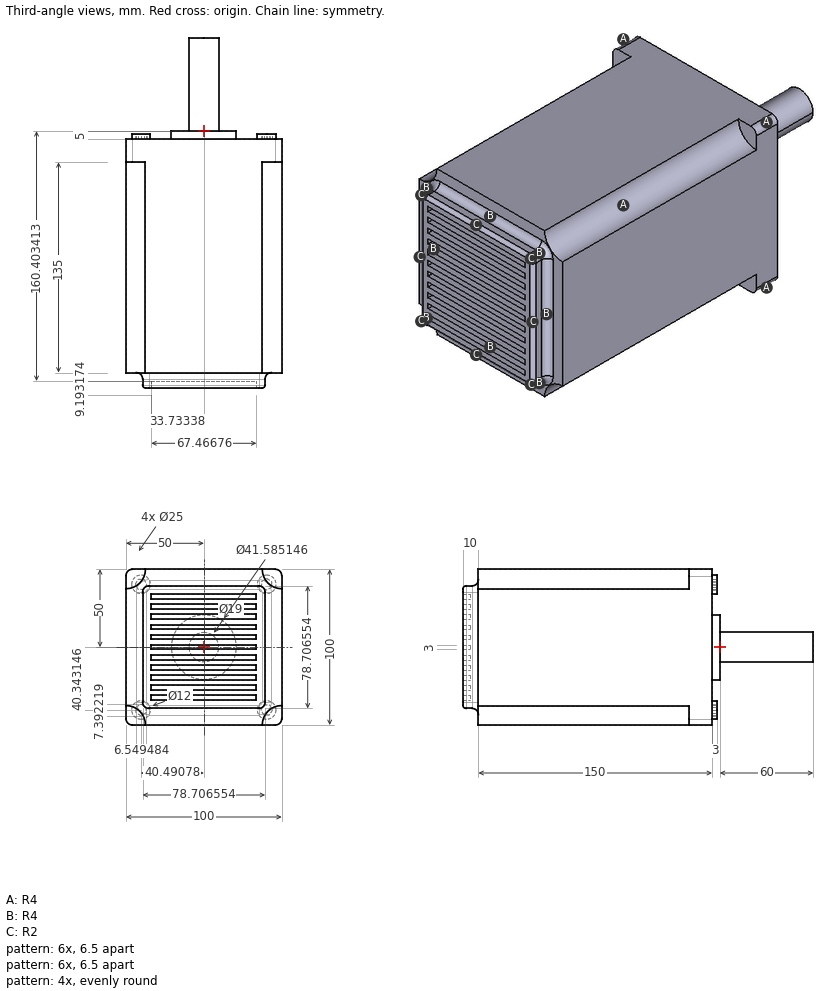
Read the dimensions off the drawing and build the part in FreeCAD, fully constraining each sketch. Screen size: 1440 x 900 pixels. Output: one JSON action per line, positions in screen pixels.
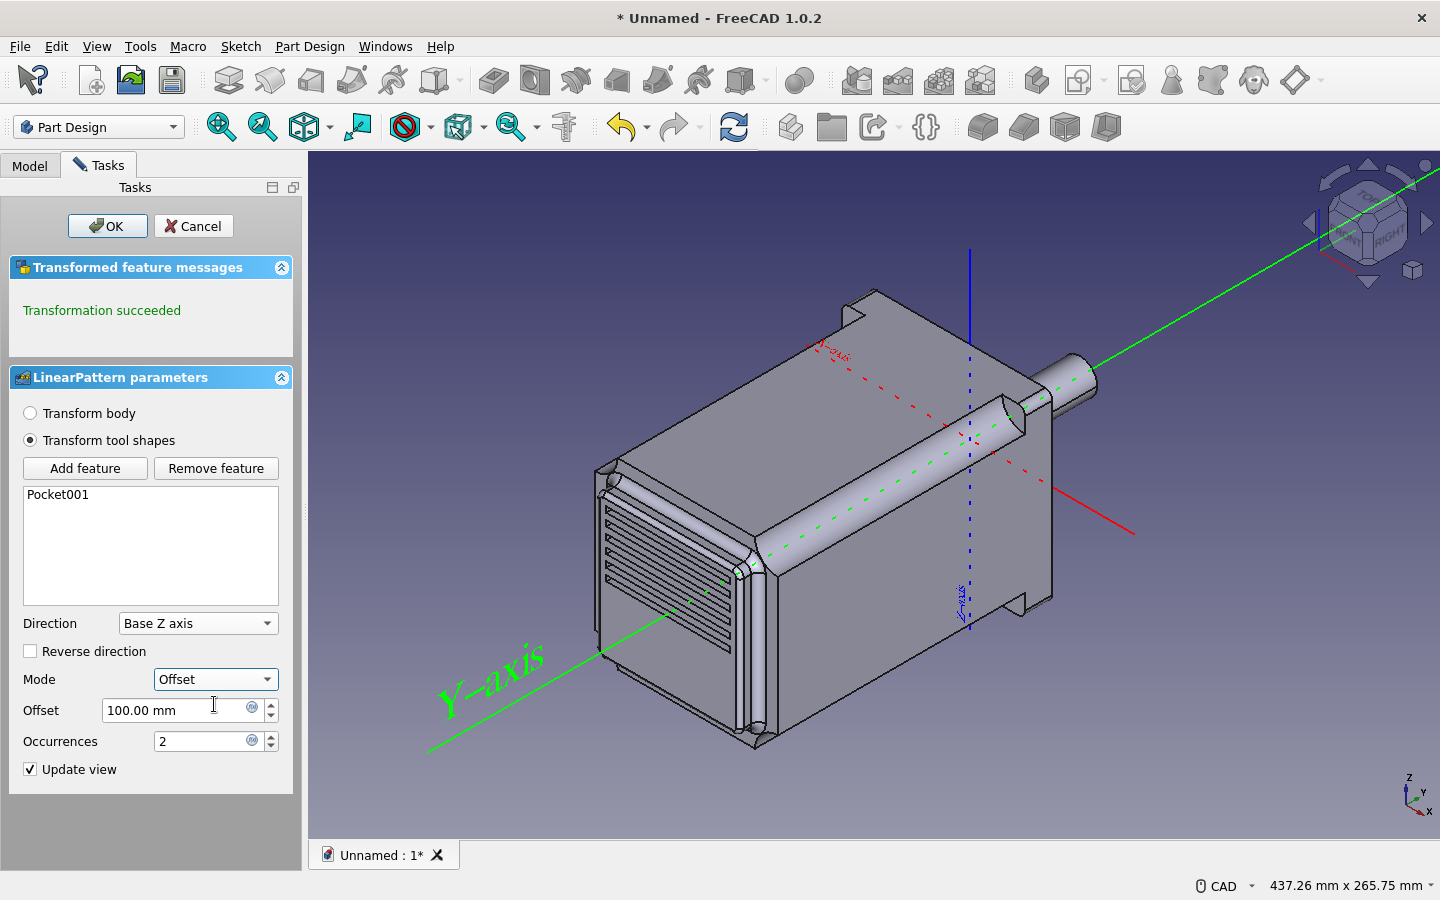
{"action": "triple_click", "coordinate": [184, 710]}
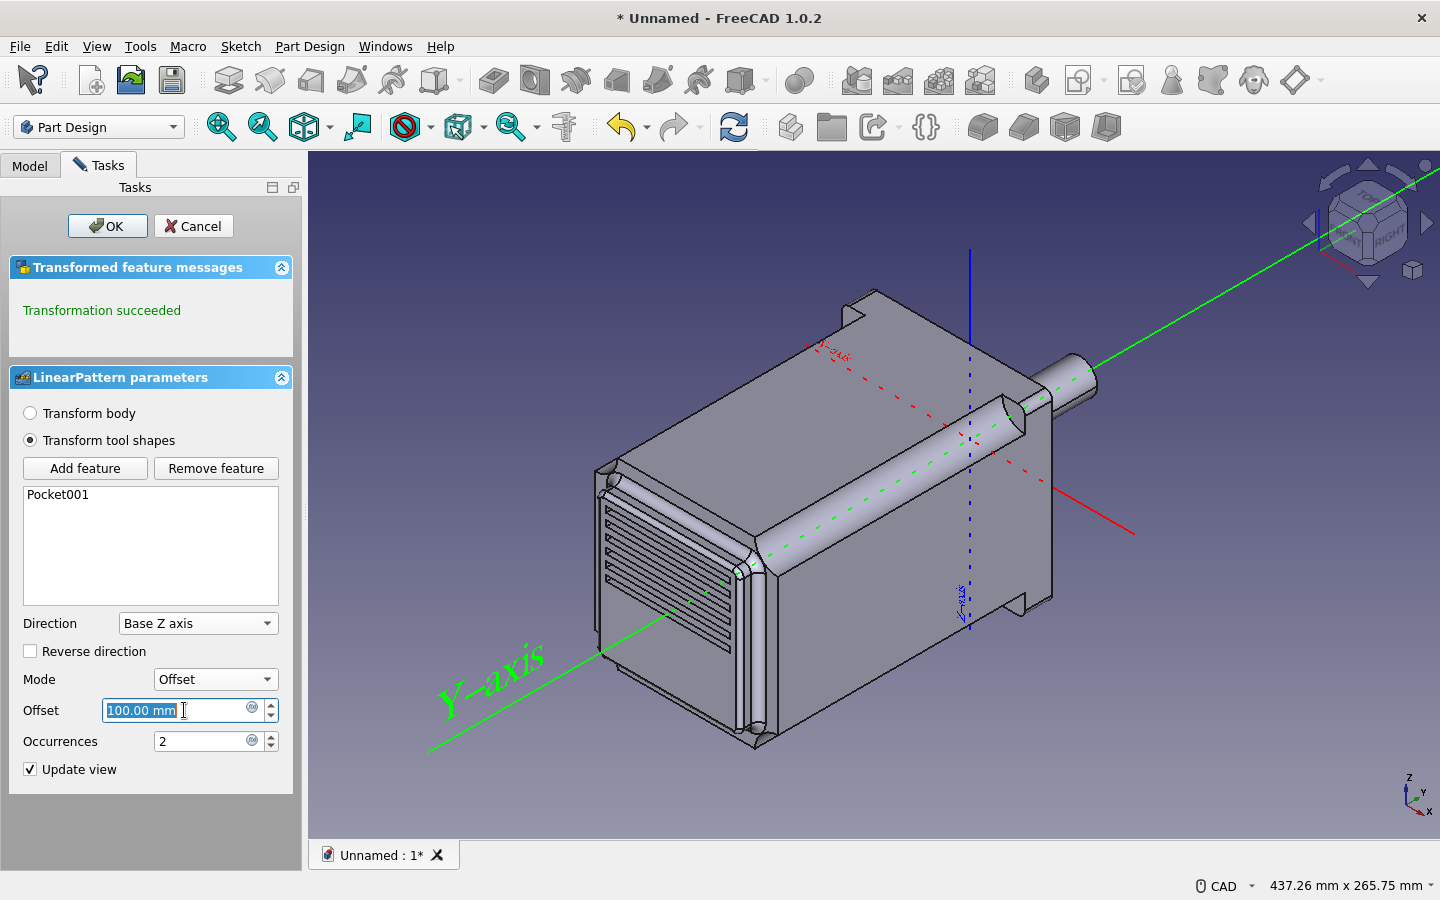
{"action": "type", "text": "6.5"}
{"action": "key", "text": "Tab"}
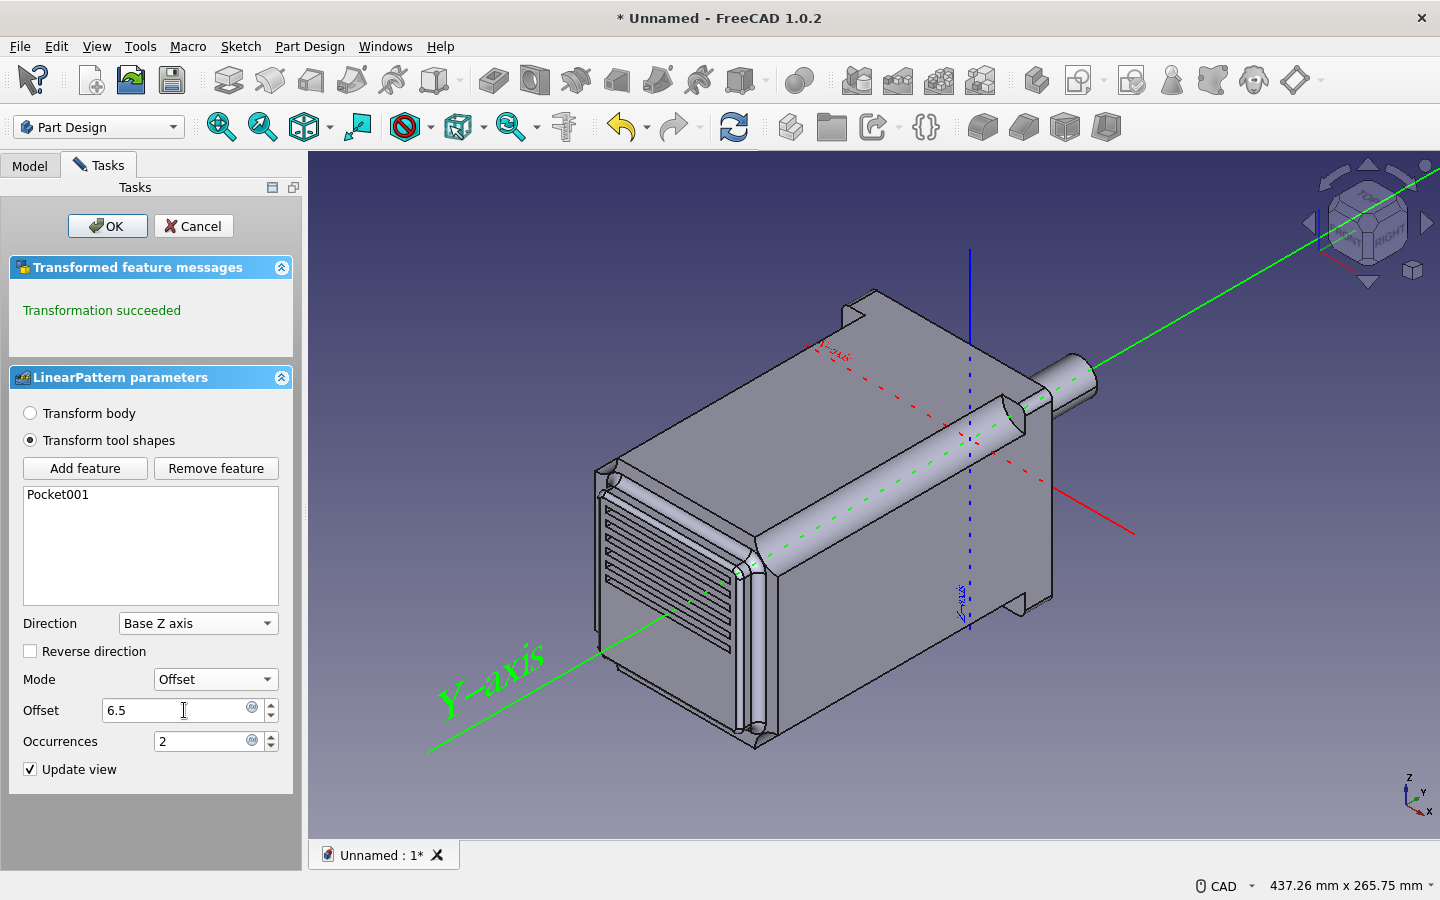
{"action": "triple_click", "coordinate": [210, 742]}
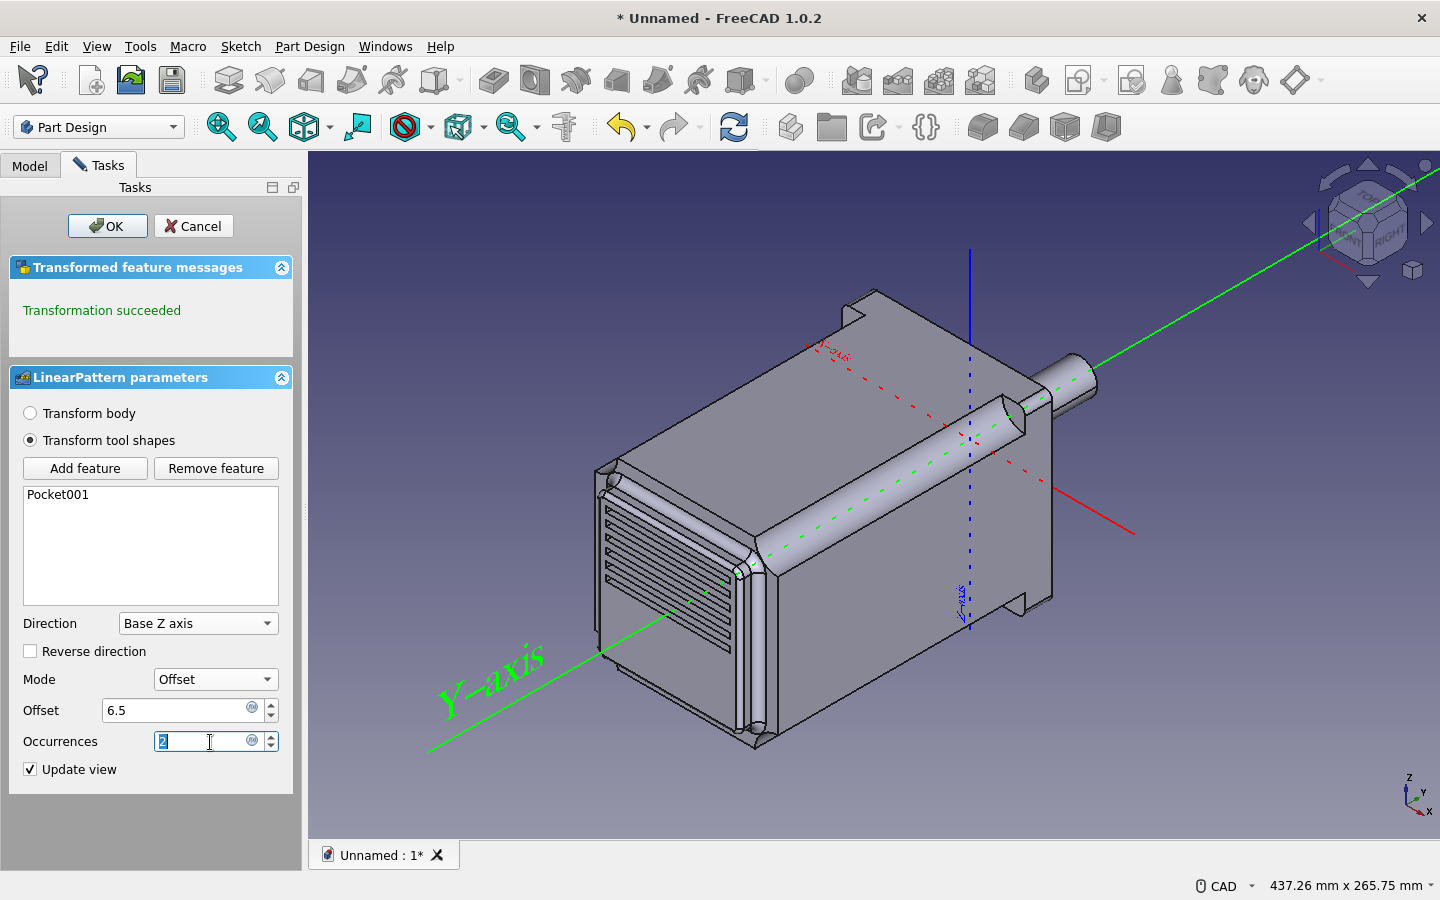
{"action": "type", "text": "6"}
{"action": "key", "text": "Tab"}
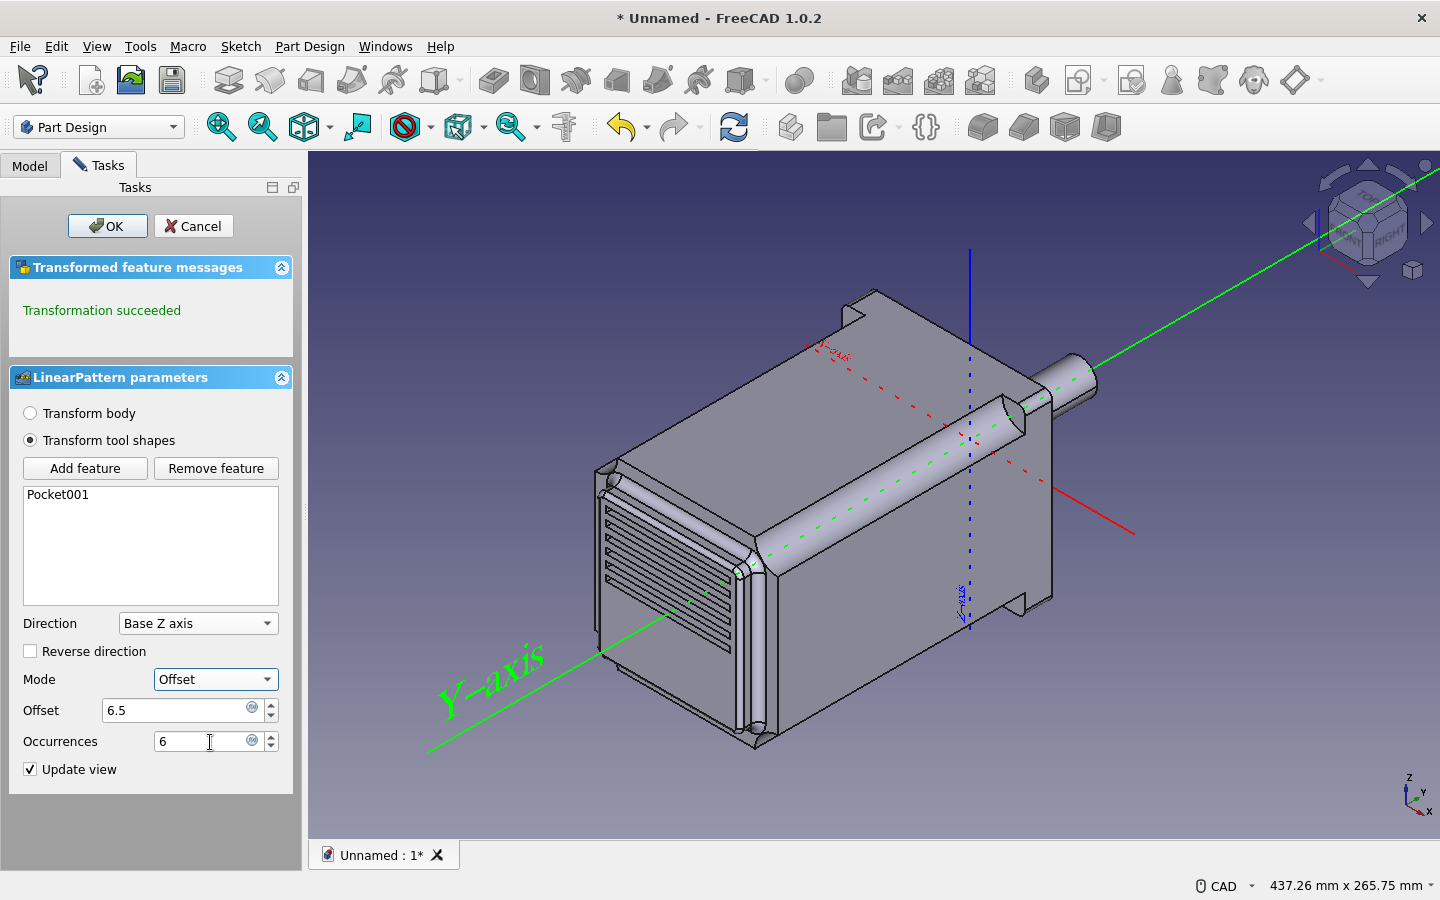
{"action": "left_click", "coordinate": [31, 651]}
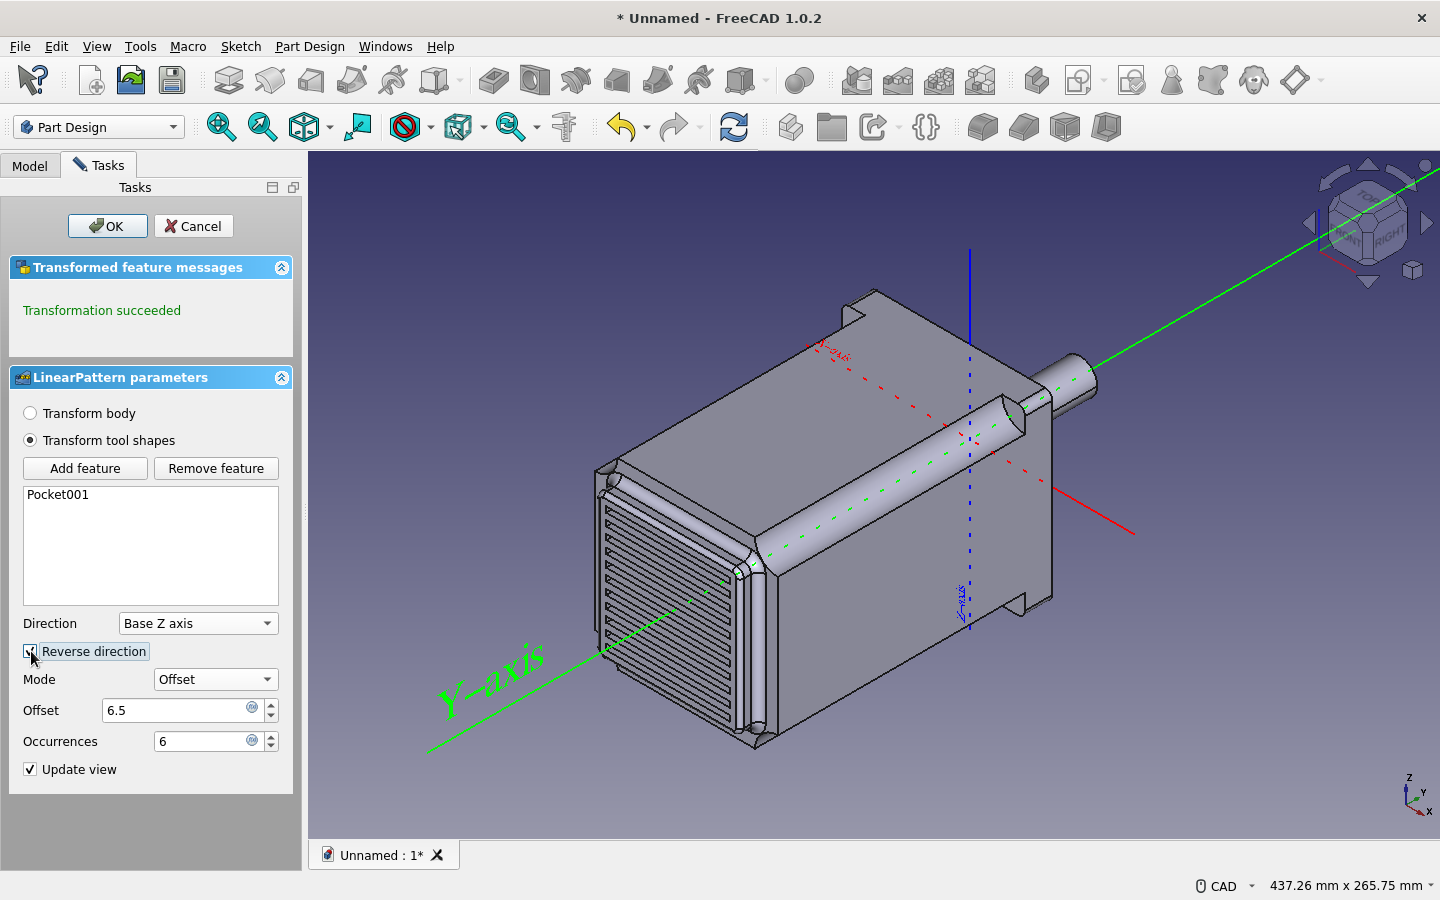
{"action": "left_click", "coordinate": [108, 226]}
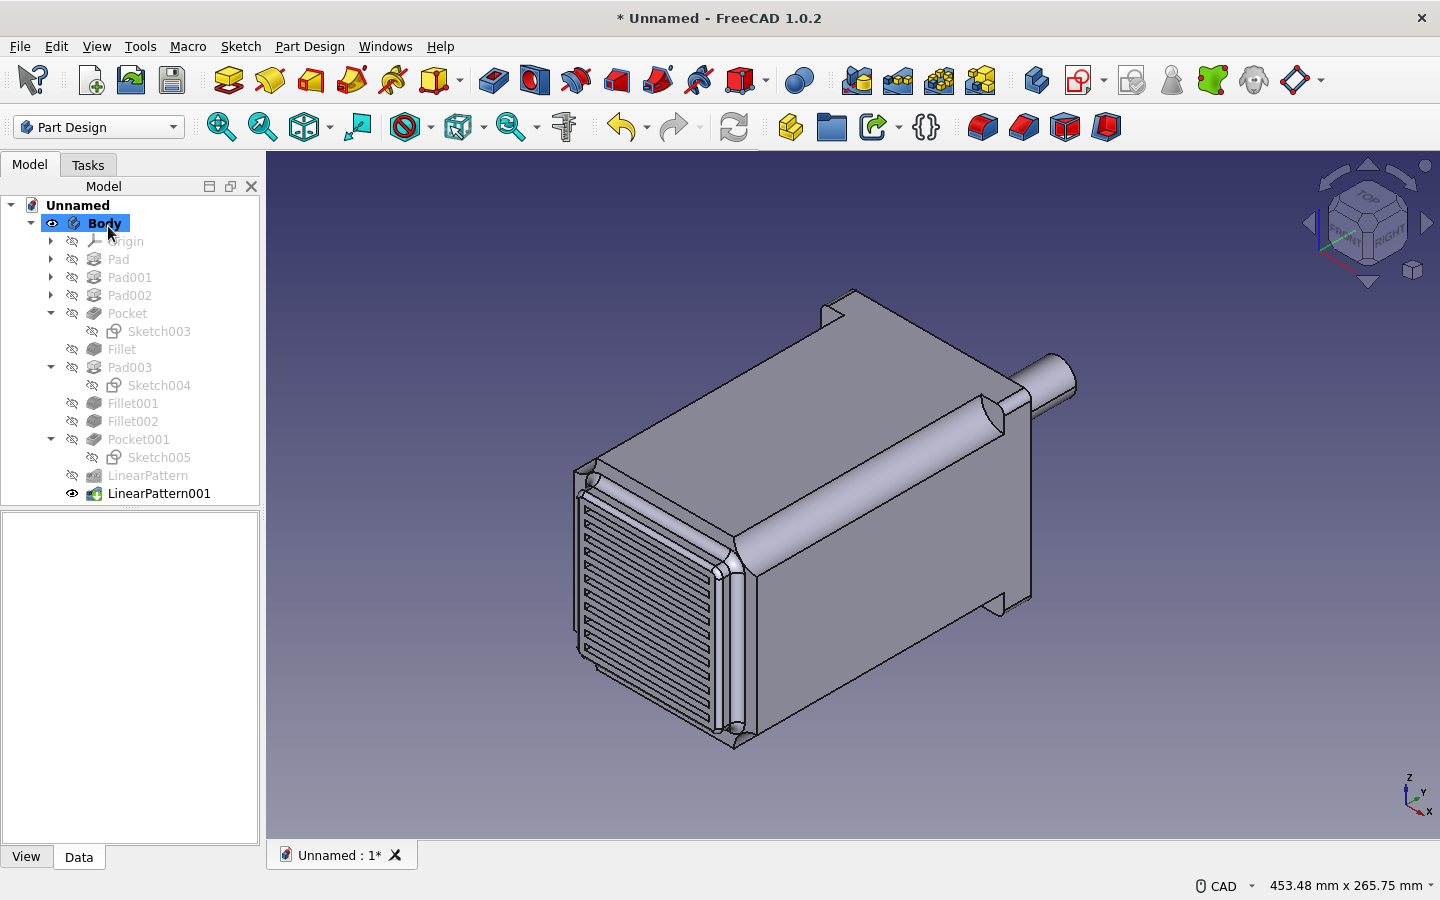
{"action": "key", "text": "4"}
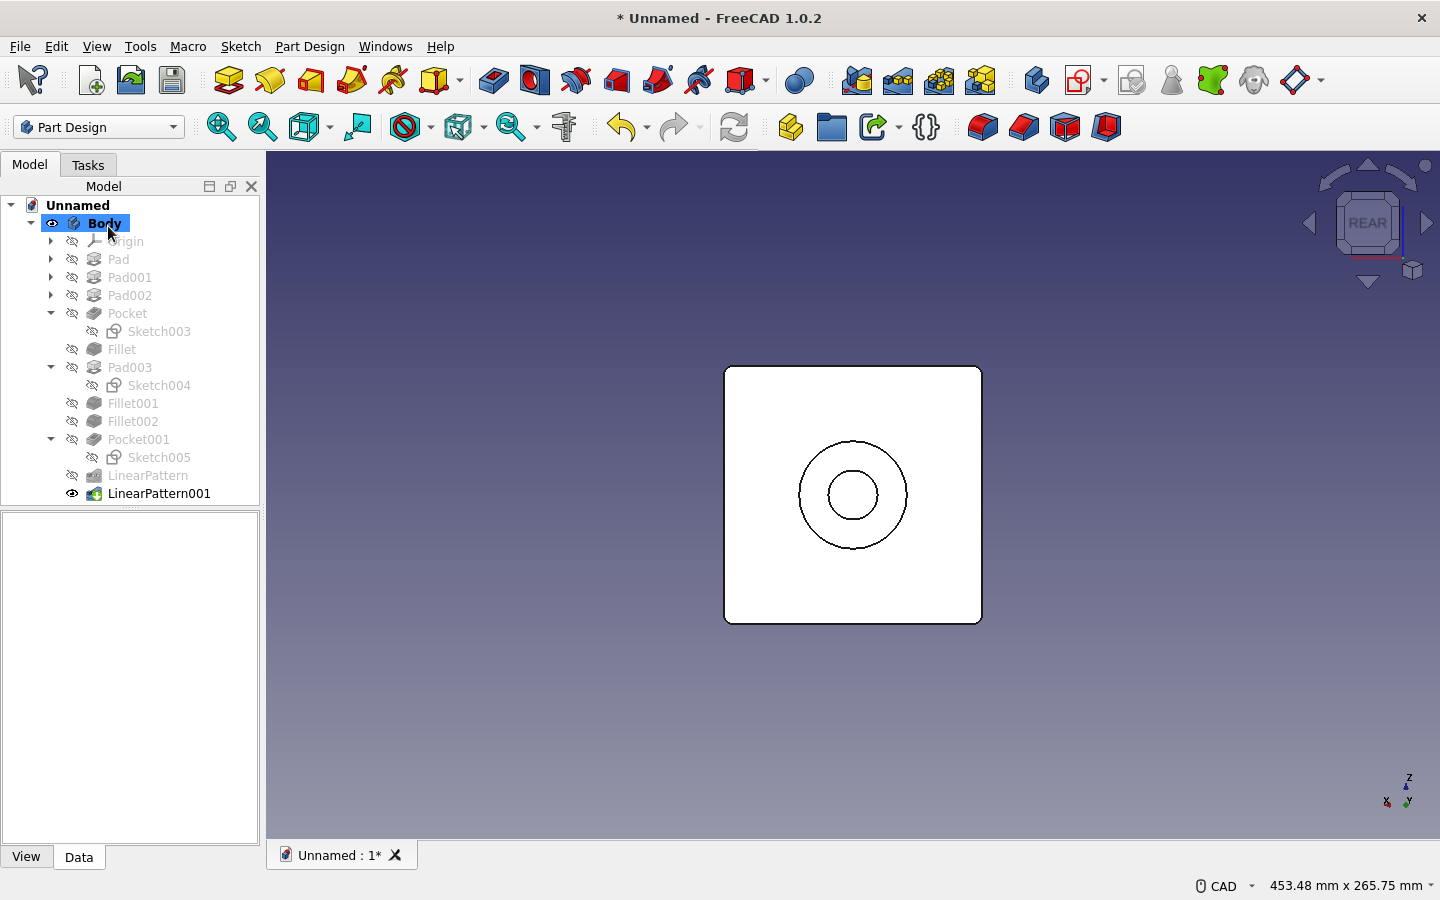
{"action": "left_click", "coordinate": [222, 128]}